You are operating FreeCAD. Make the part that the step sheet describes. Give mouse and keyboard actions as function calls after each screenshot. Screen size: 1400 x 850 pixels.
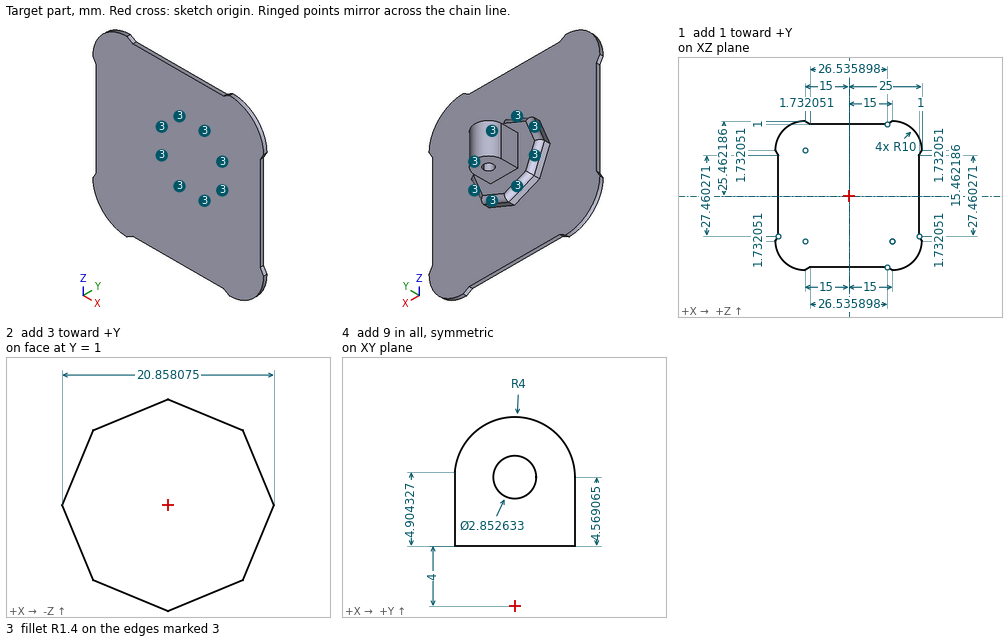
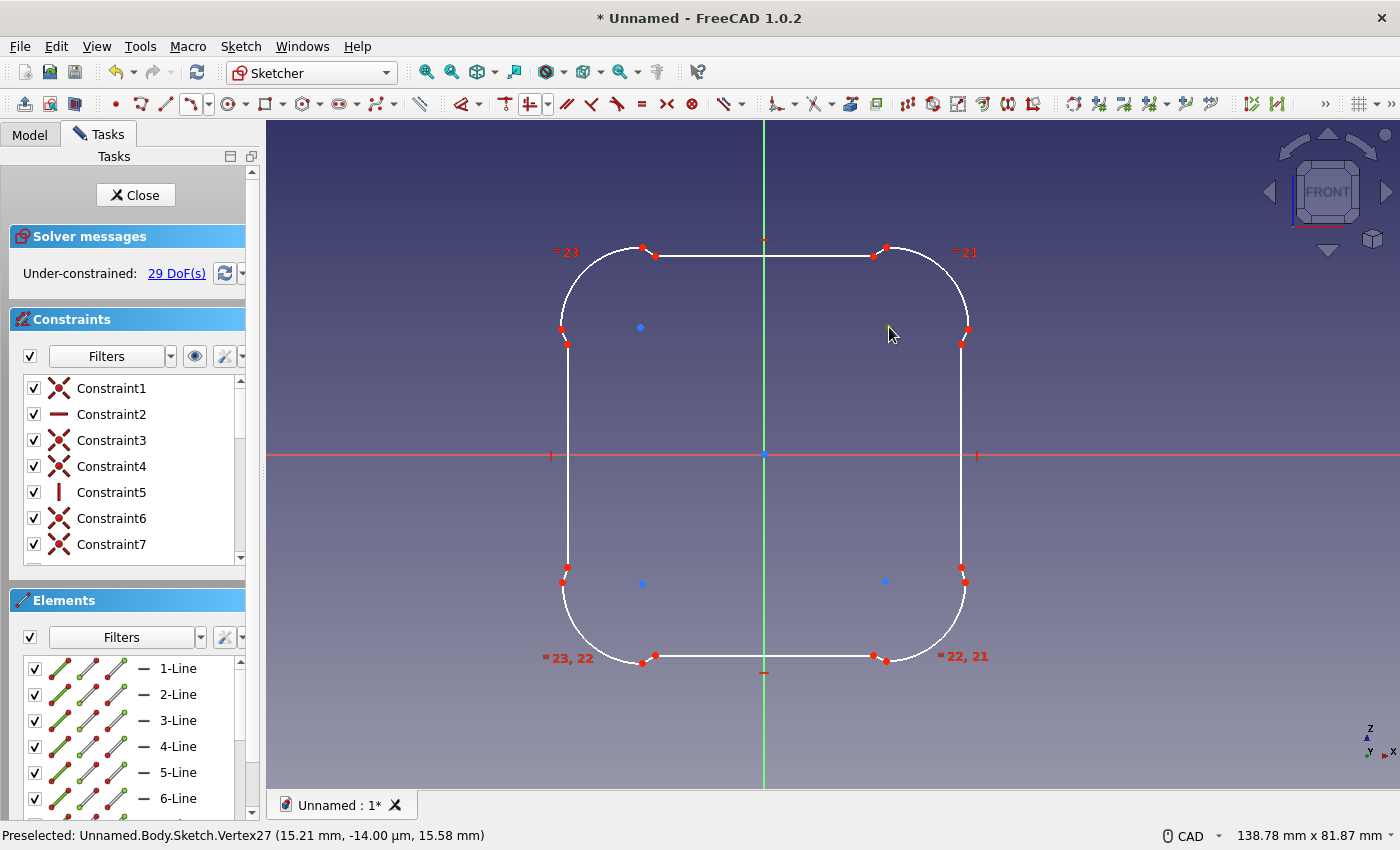
click(886, 582)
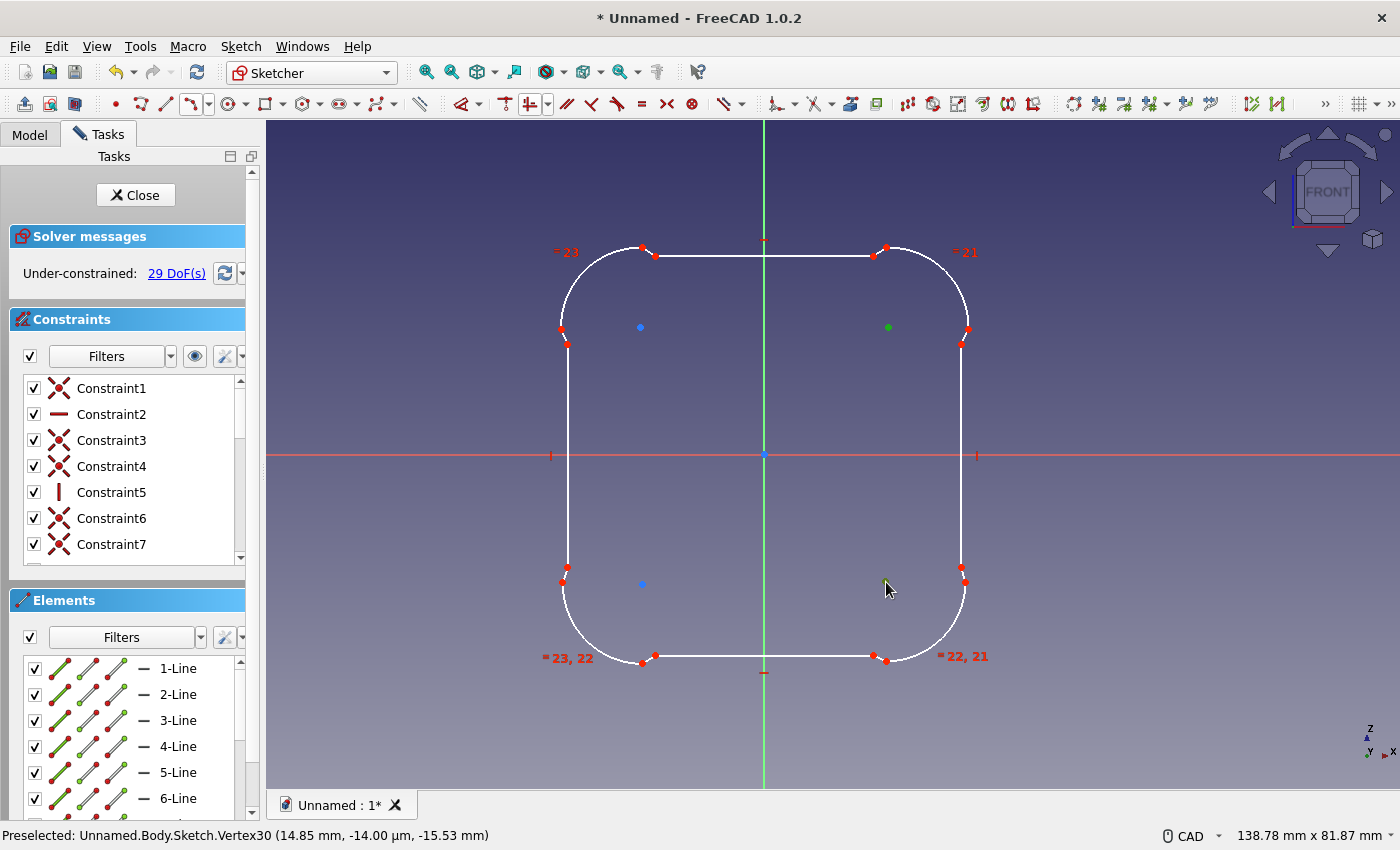
click(361, 455)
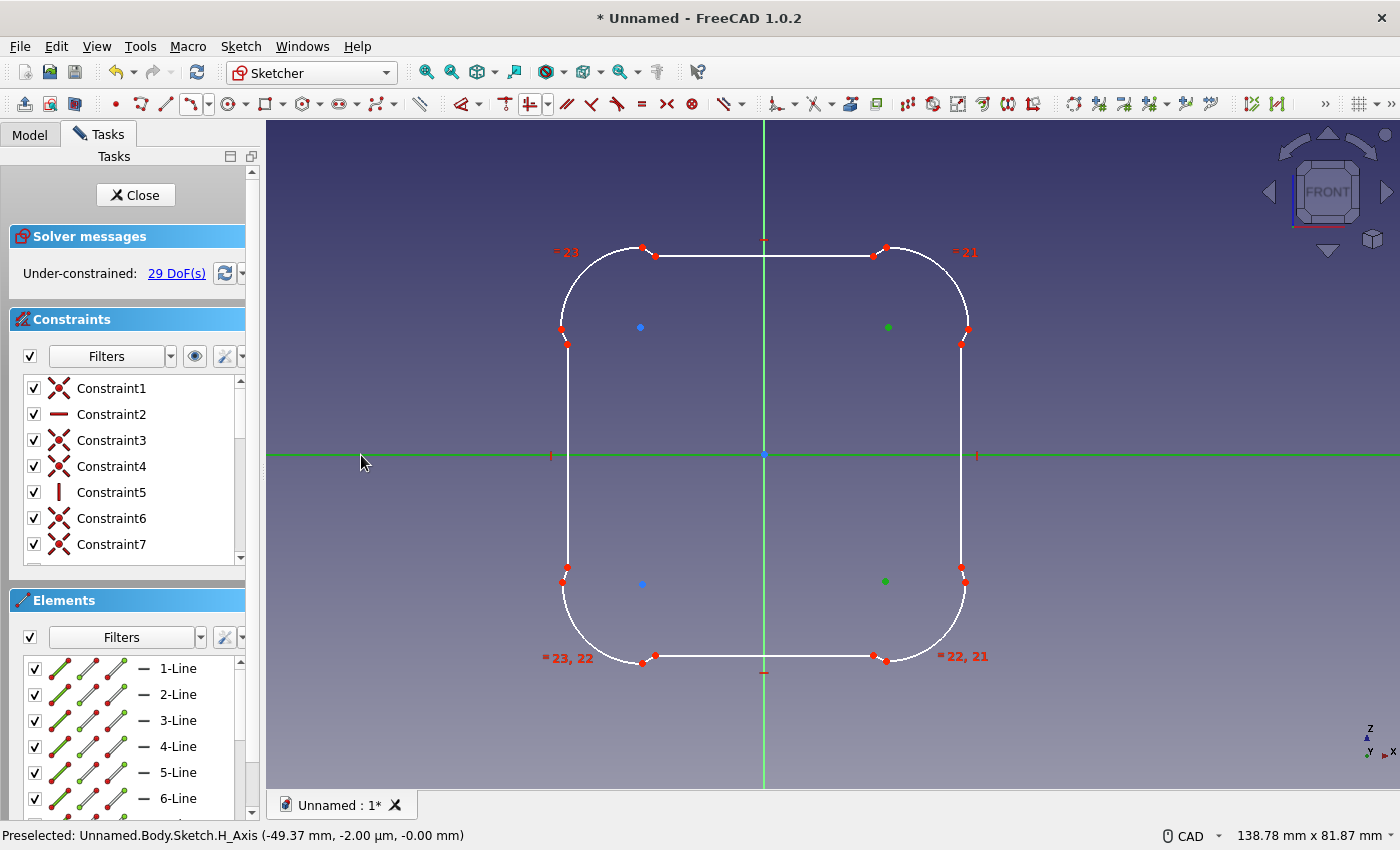
click(667, 104)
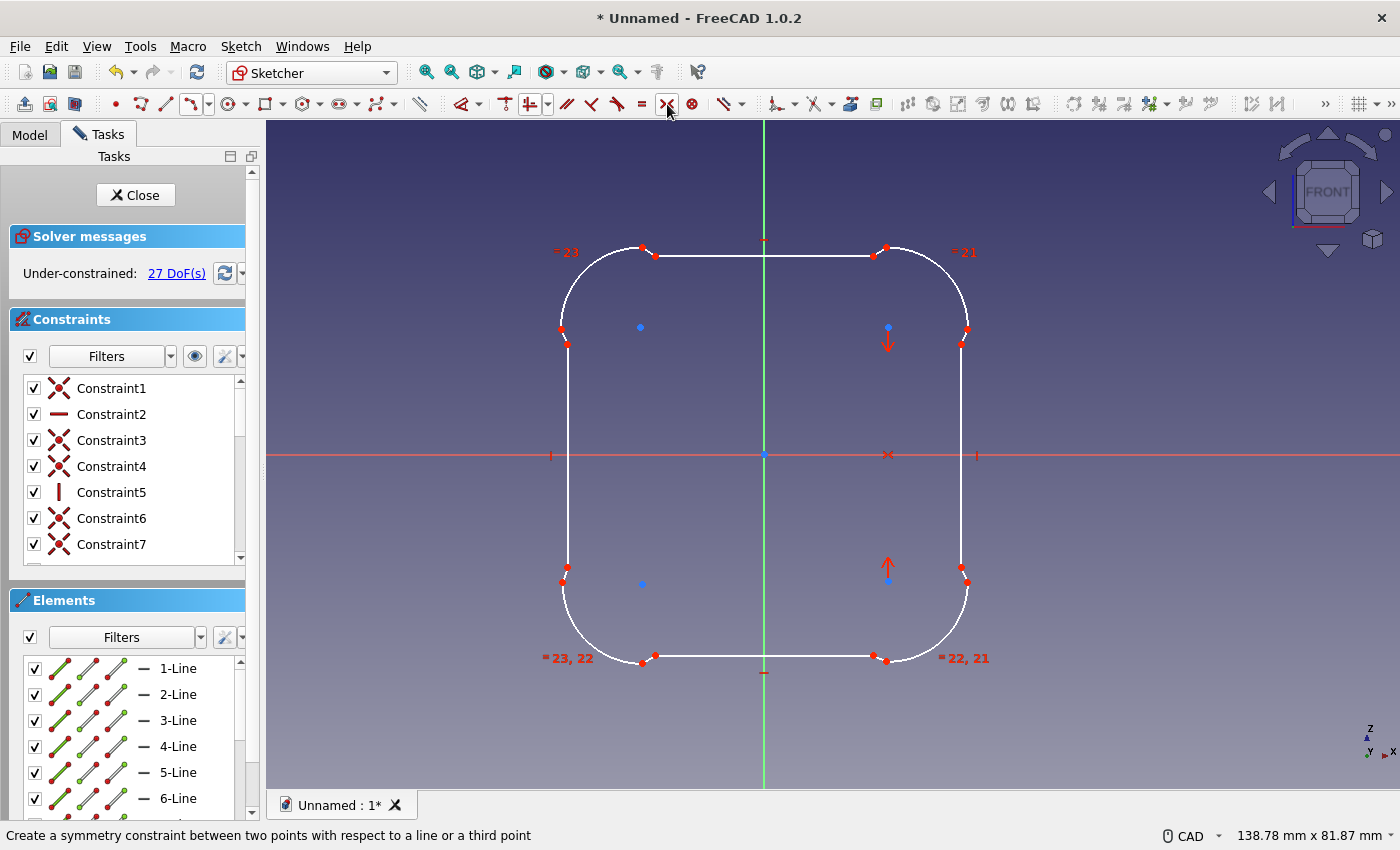
click(888, 582)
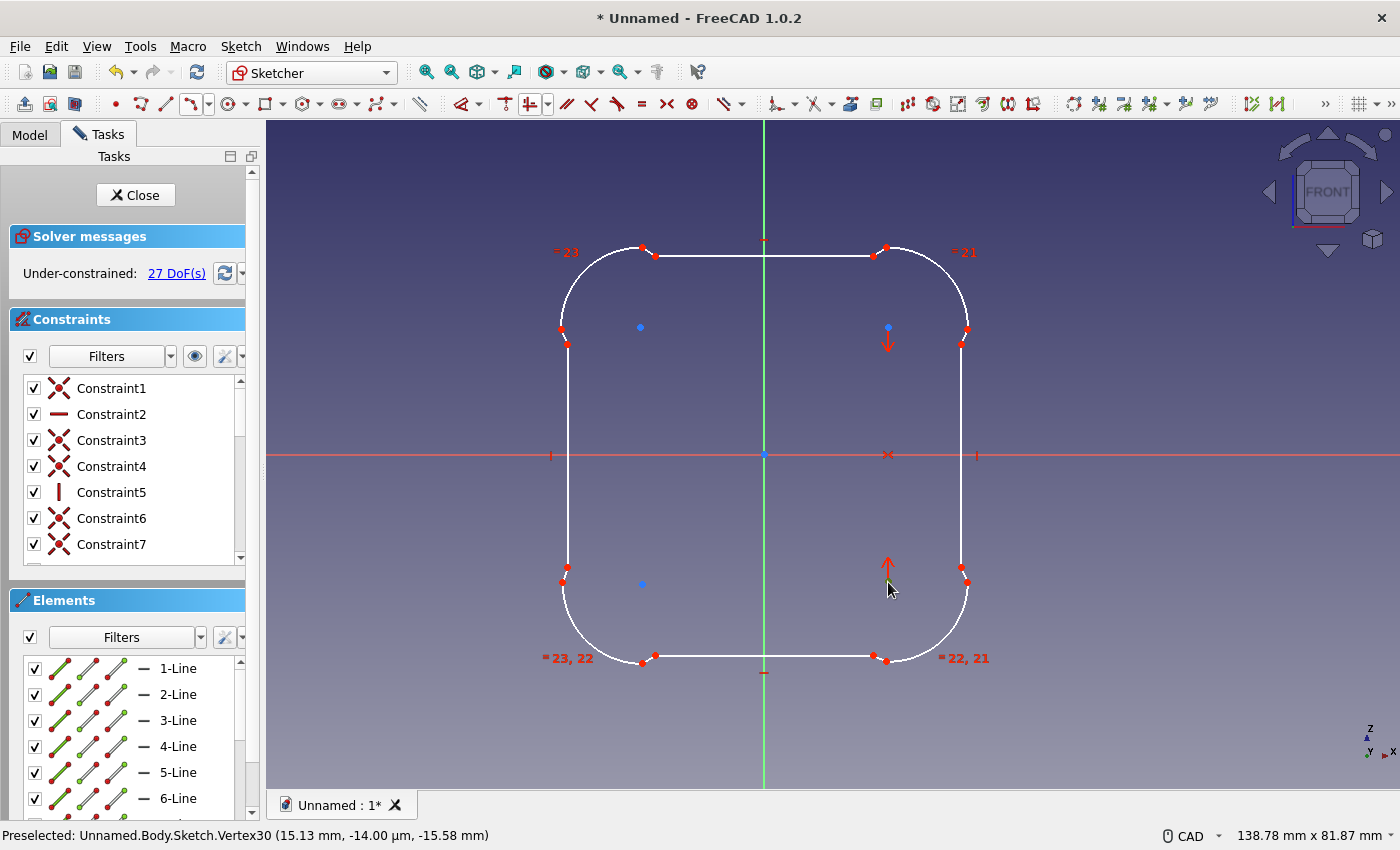
click(643, 584)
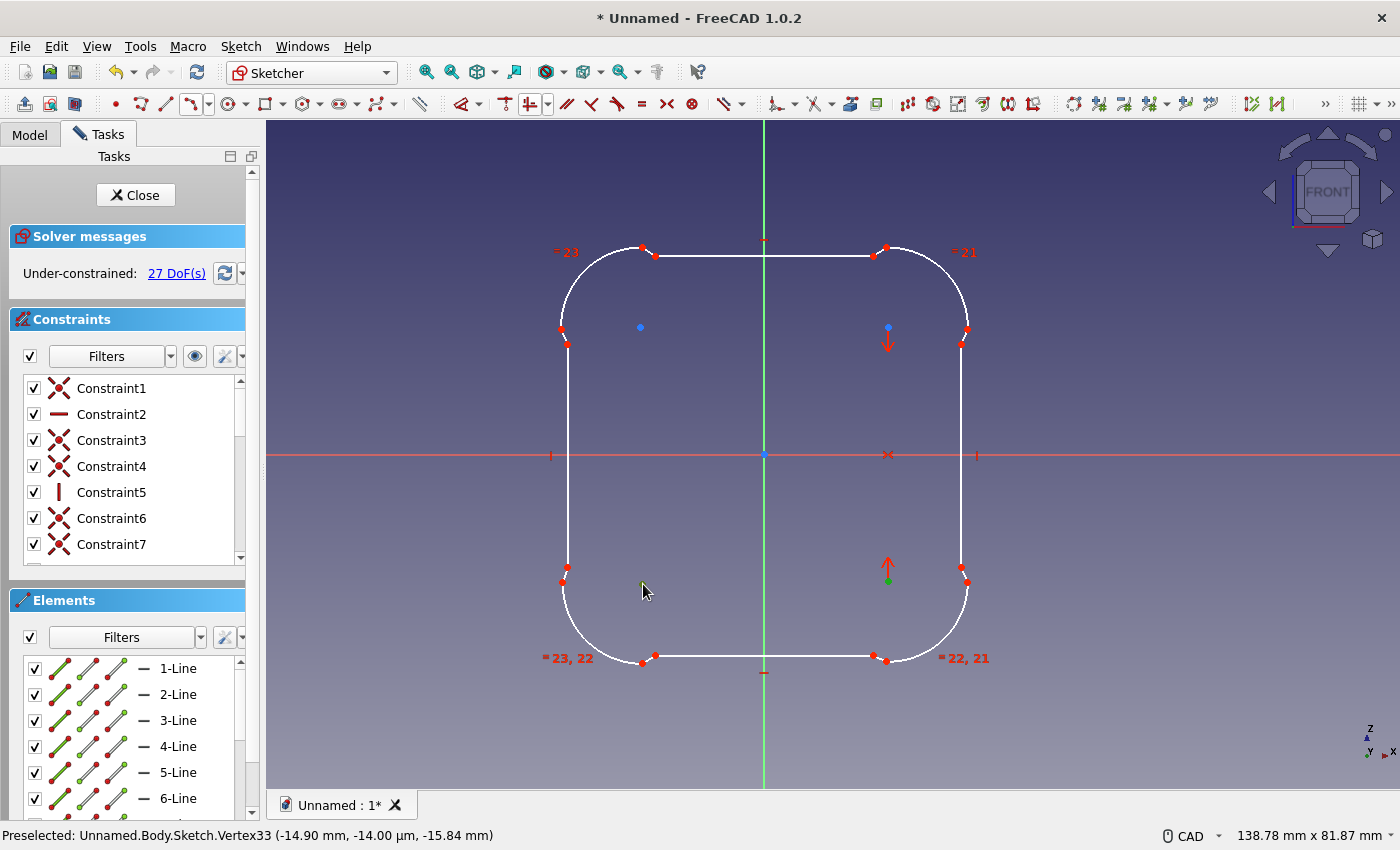
click(764, 717)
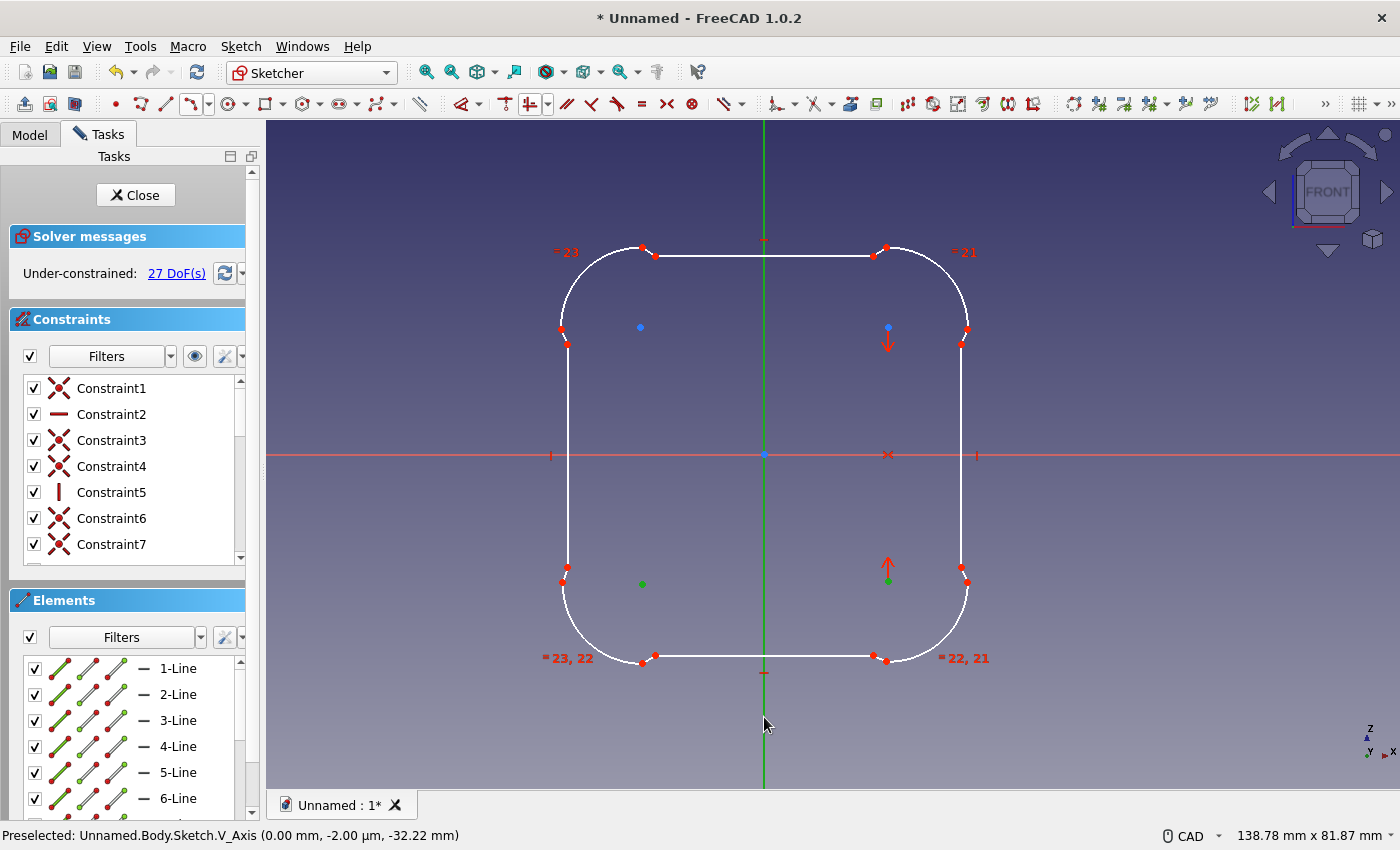
click(667, 104)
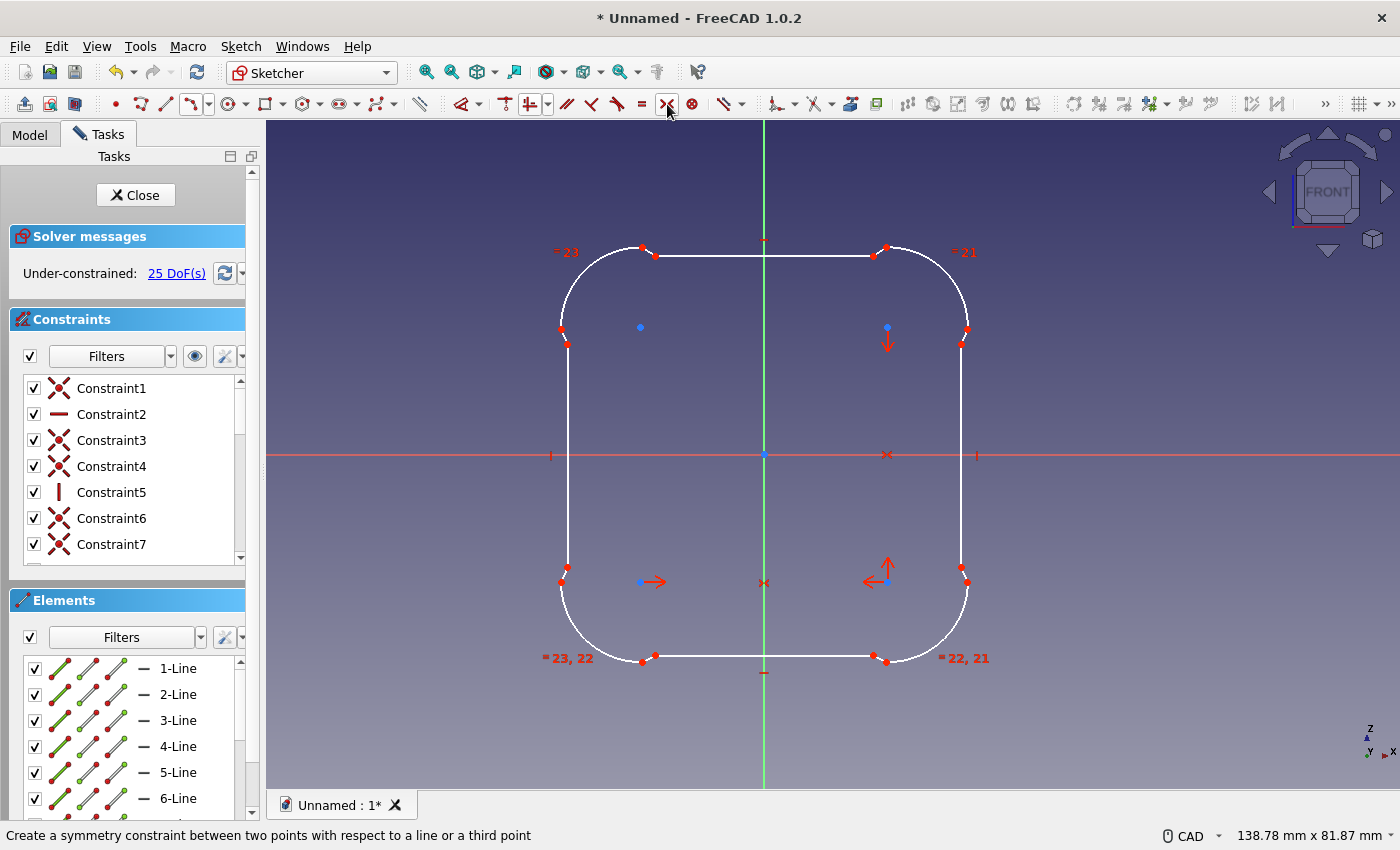
click(888, 327)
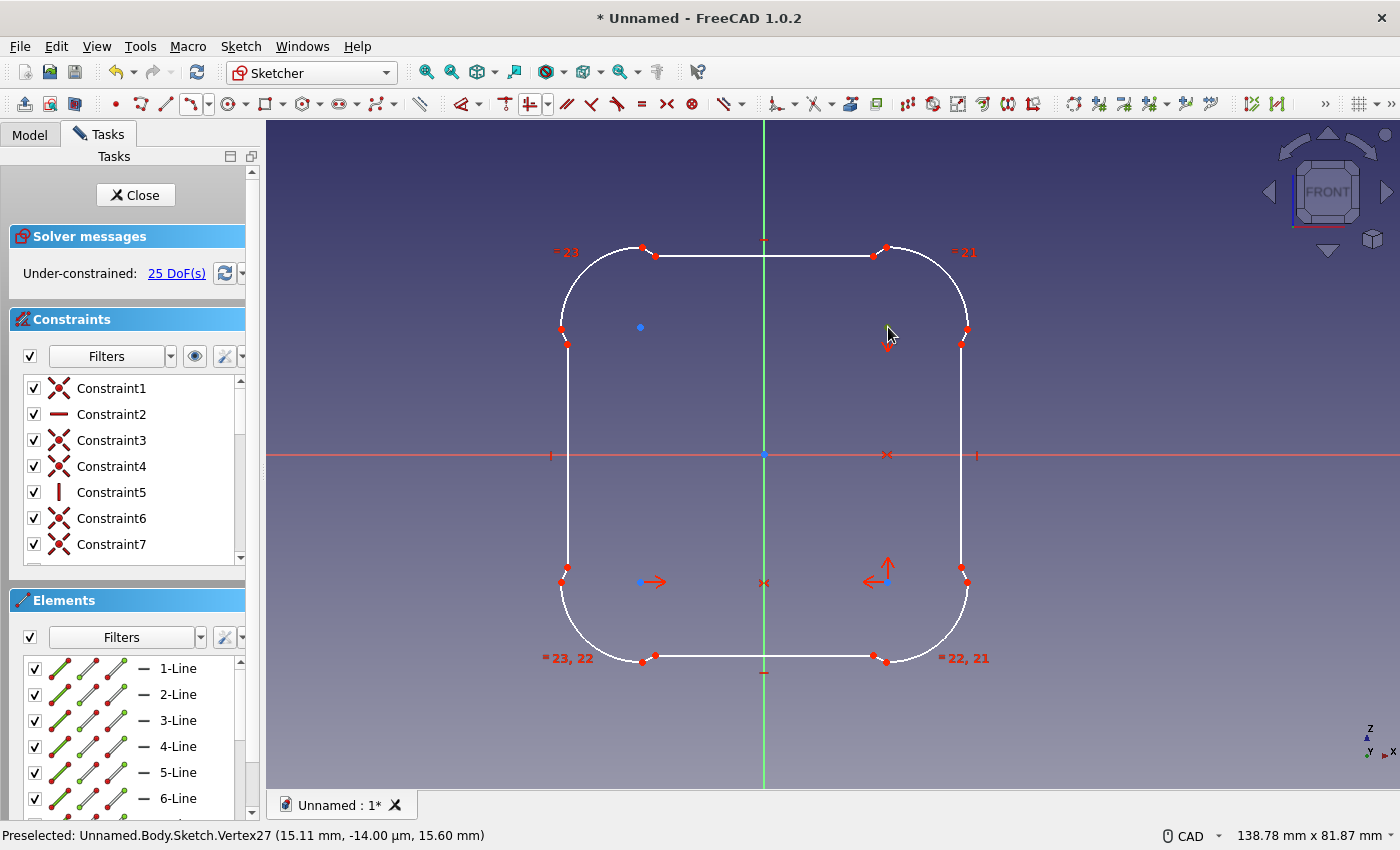
click(641, 327)